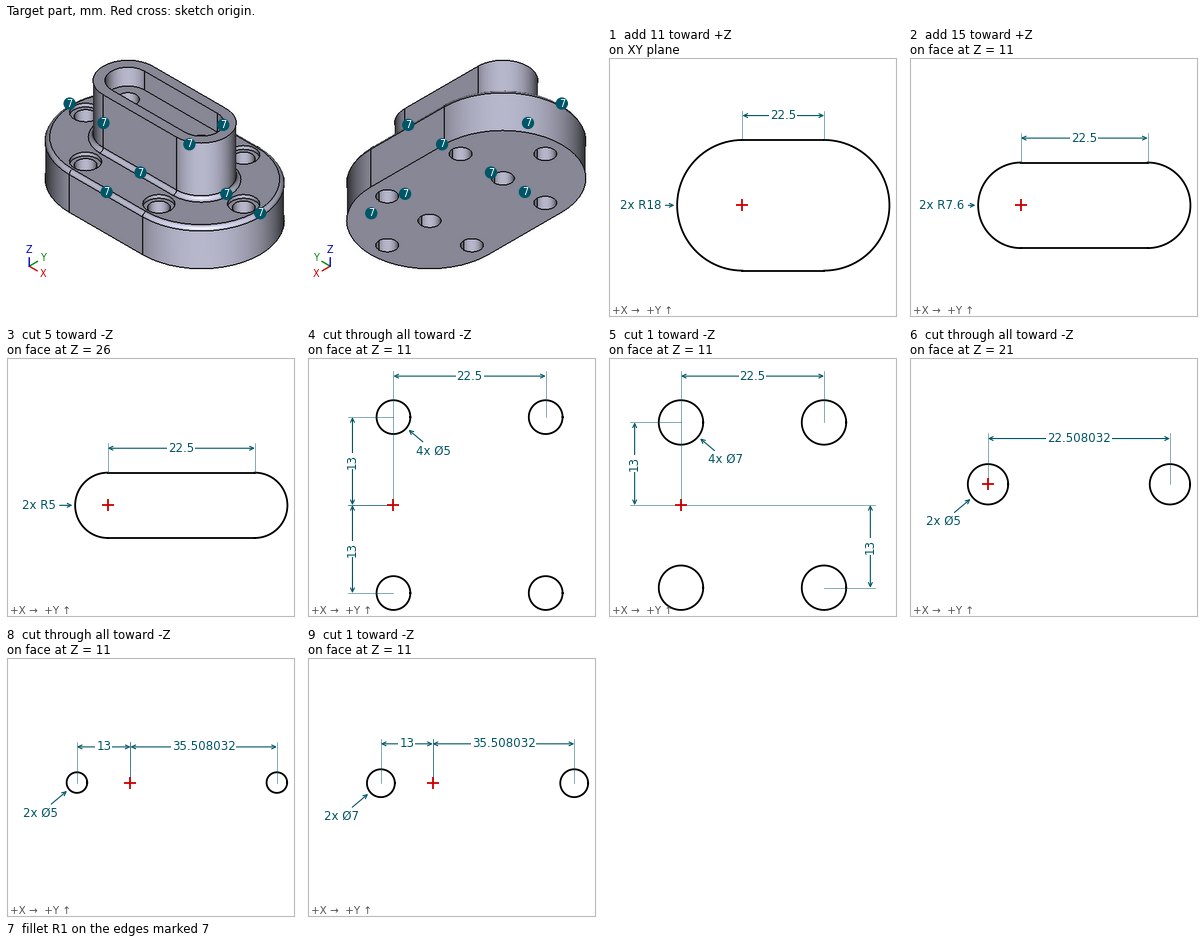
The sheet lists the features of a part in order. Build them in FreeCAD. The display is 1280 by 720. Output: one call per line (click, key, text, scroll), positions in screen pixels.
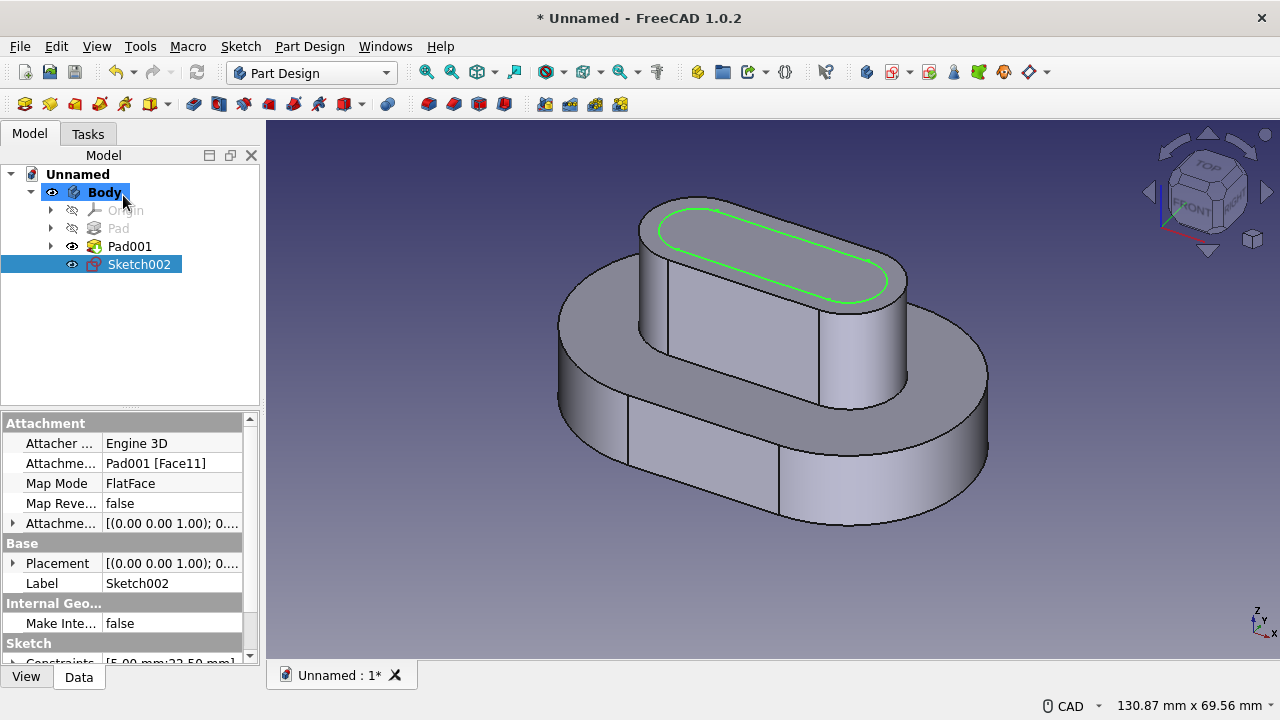
click(194, 104)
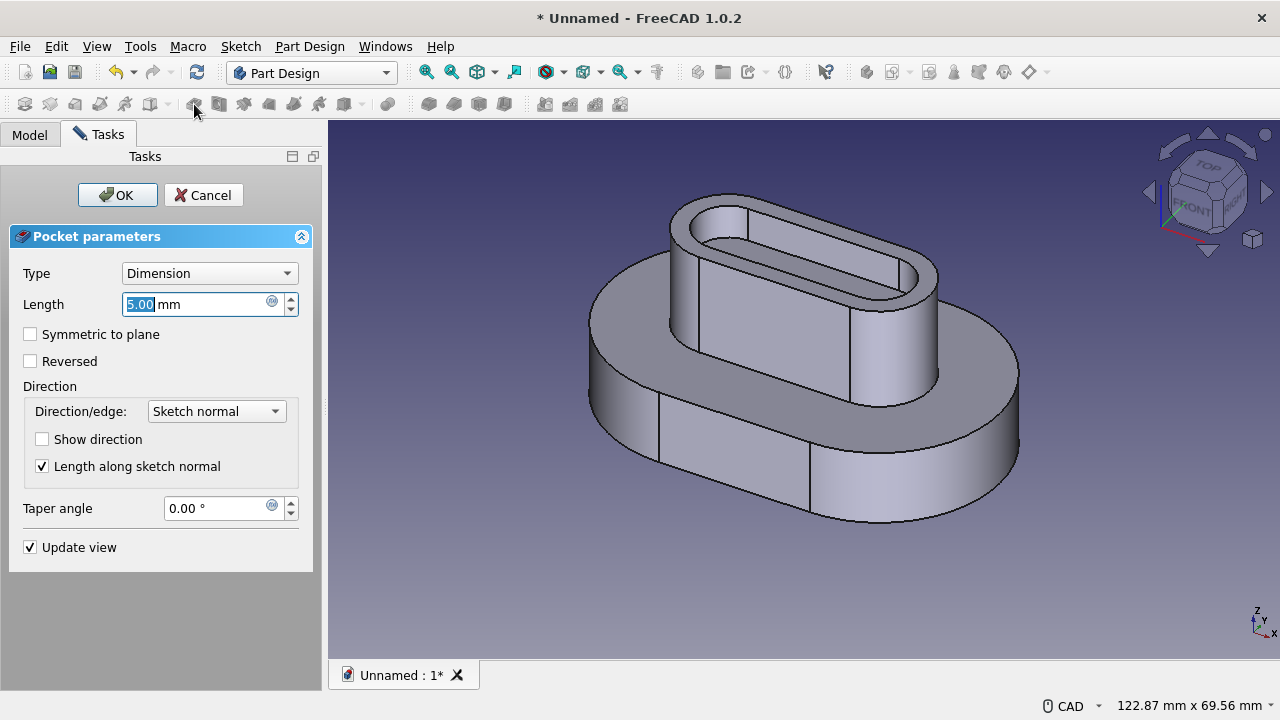
text(5)
key(Tab)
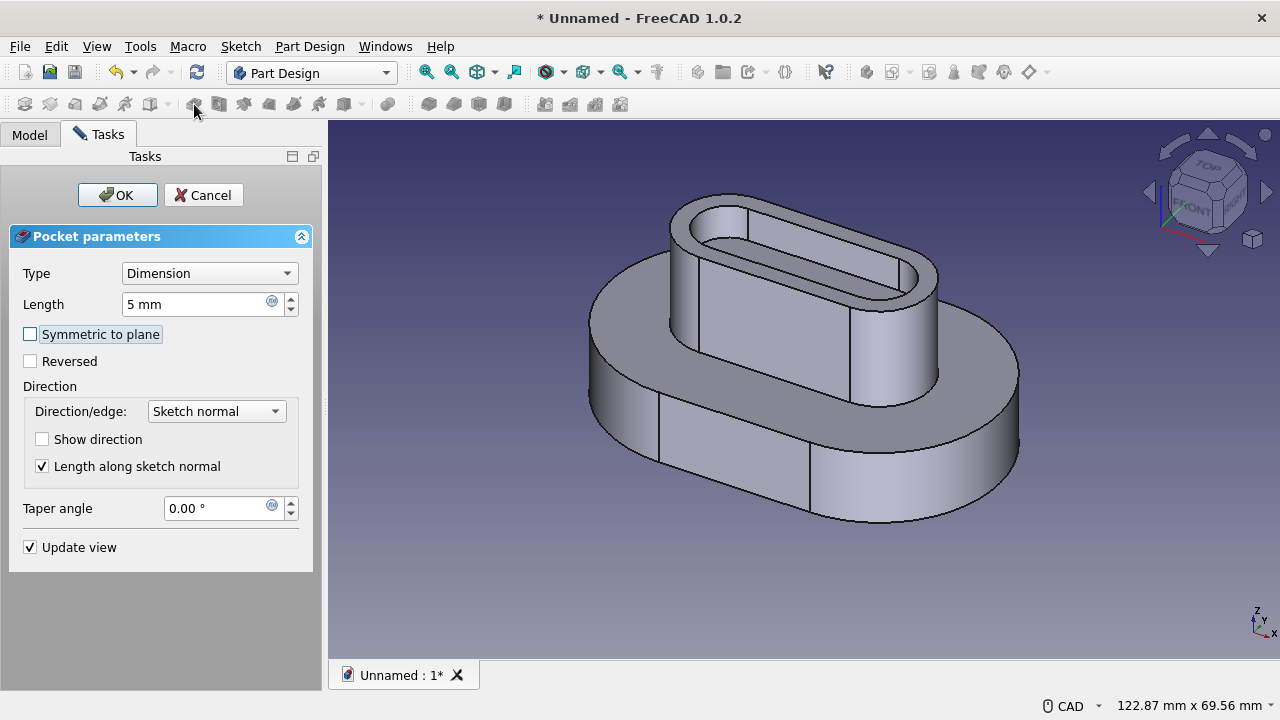
click(118, 195)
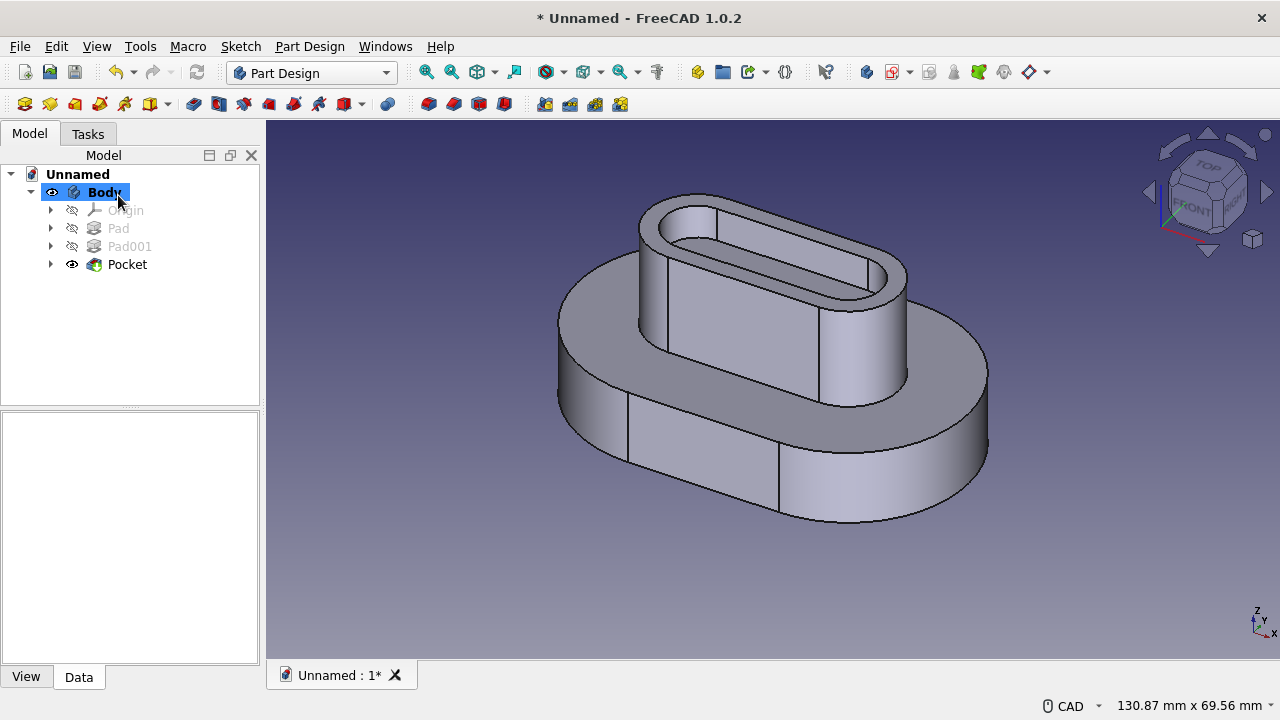
key(v)
key(f)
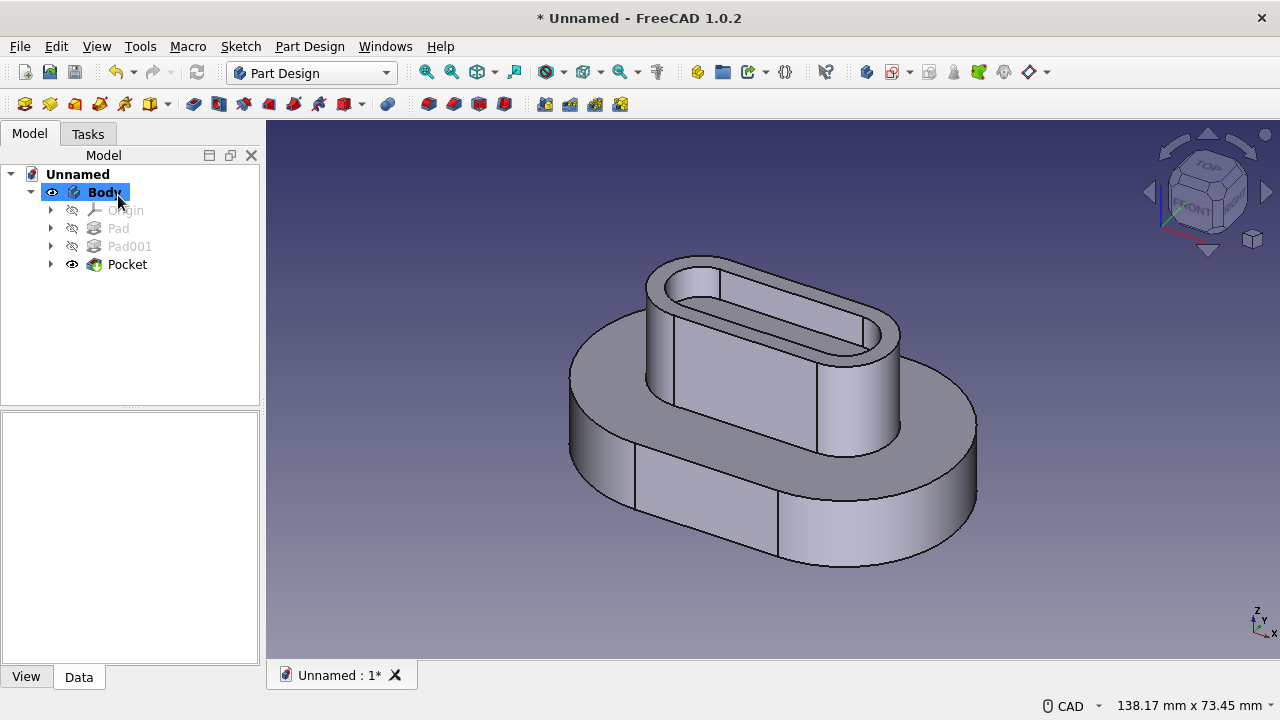
click(932, 453)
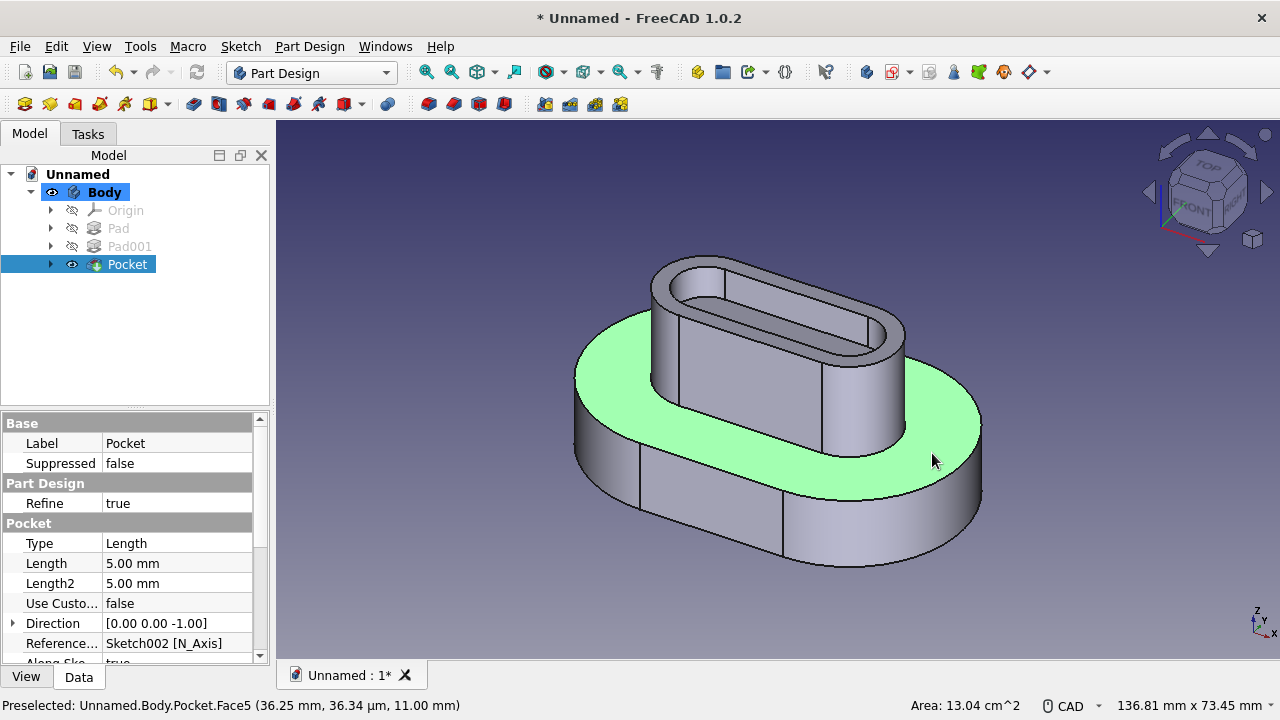
click(892, 72)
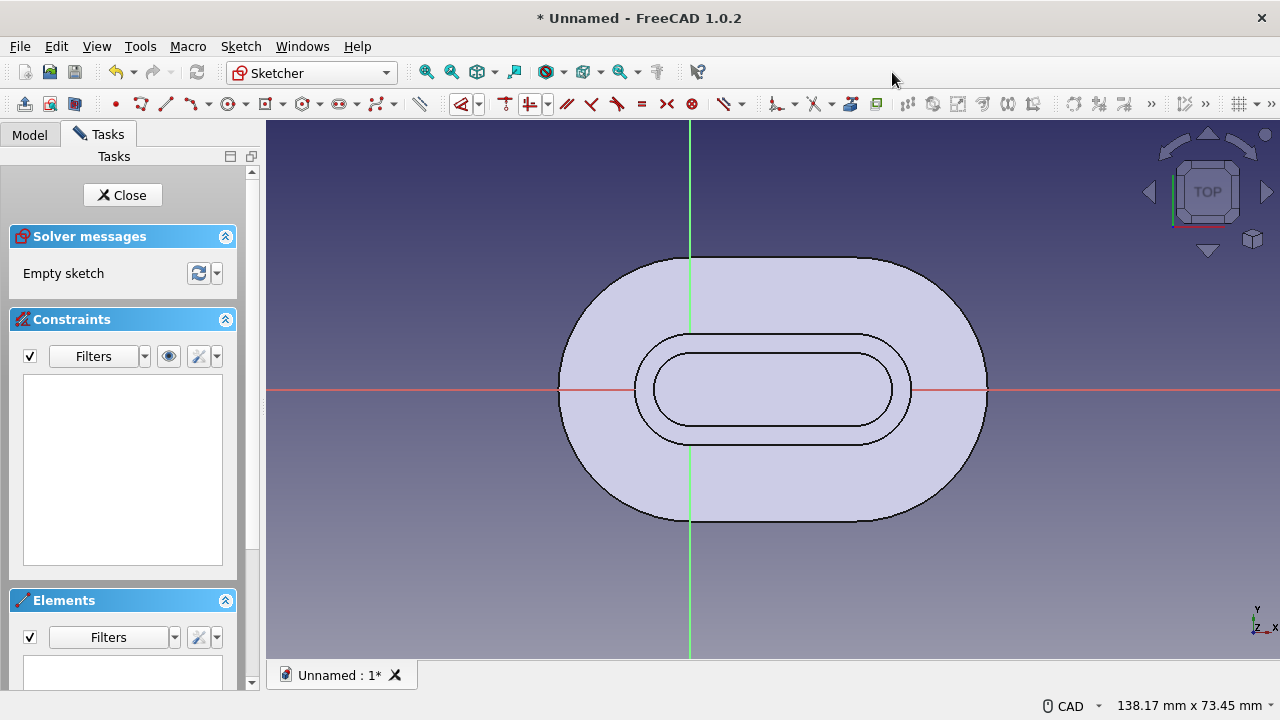
scroll(912, 390, up, 2)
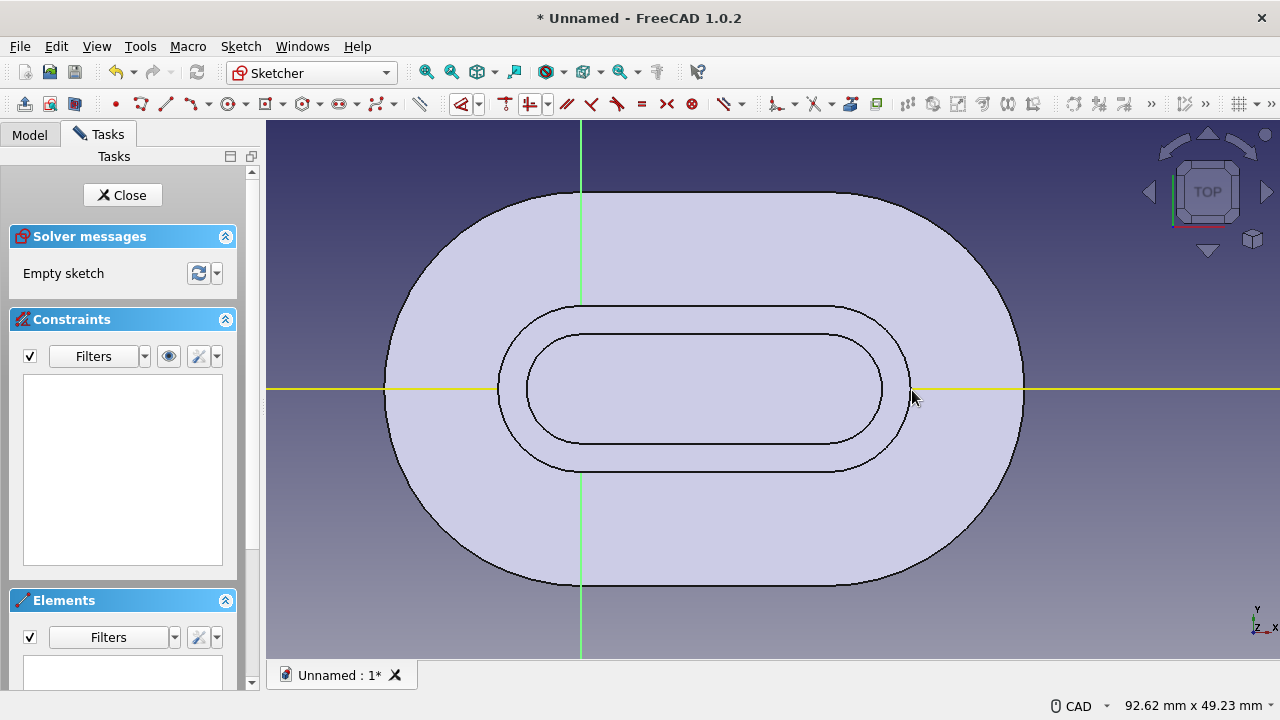
key(g)
key(c)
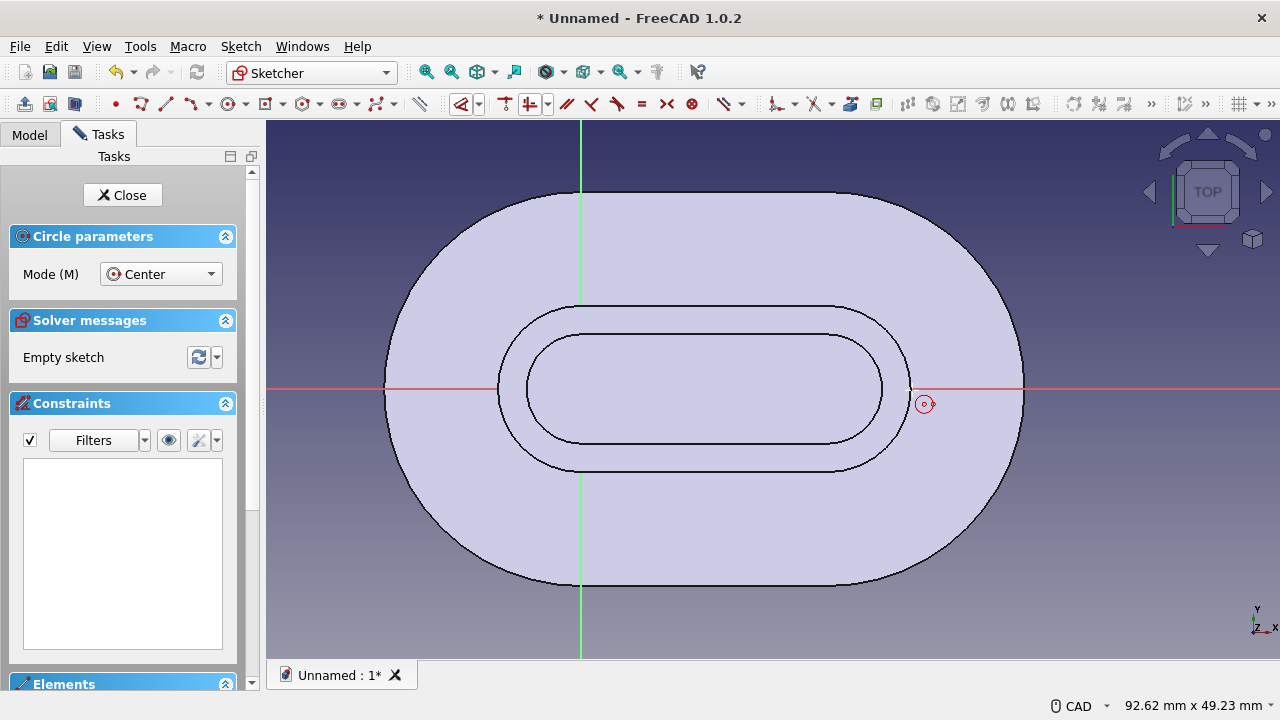
click(581, 247)
move(601, 227)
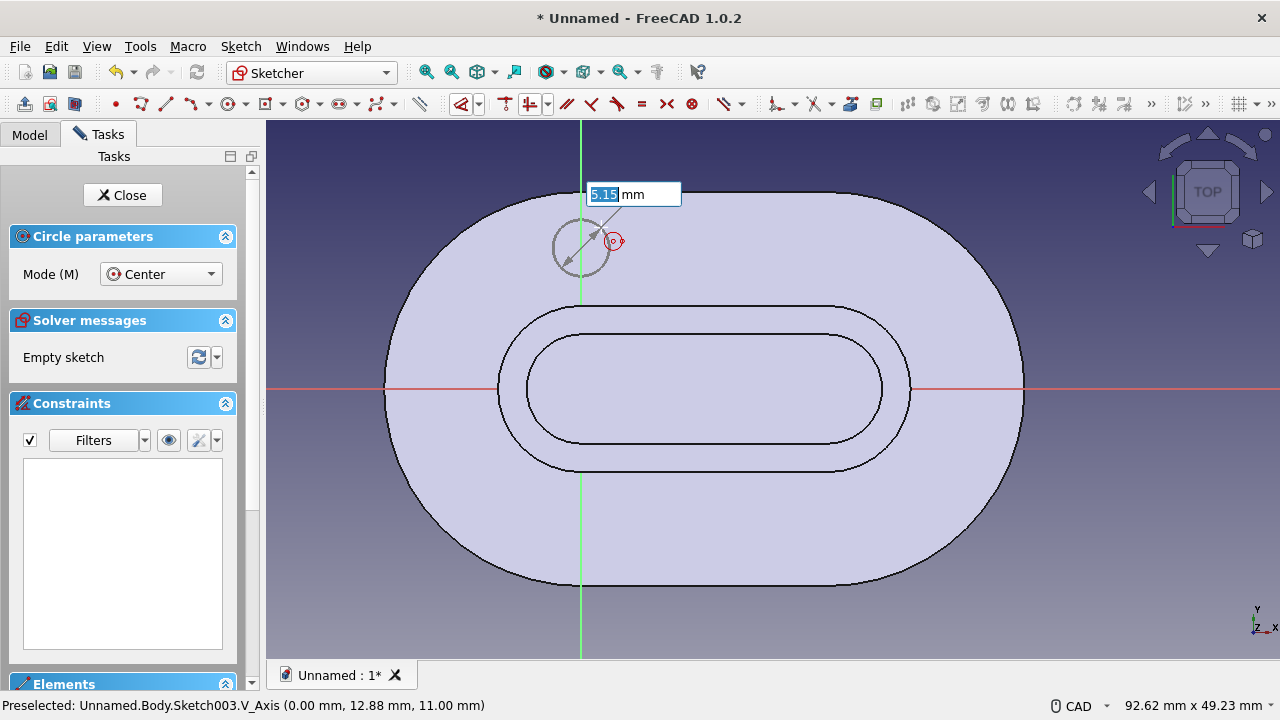
text(5)
key(Return)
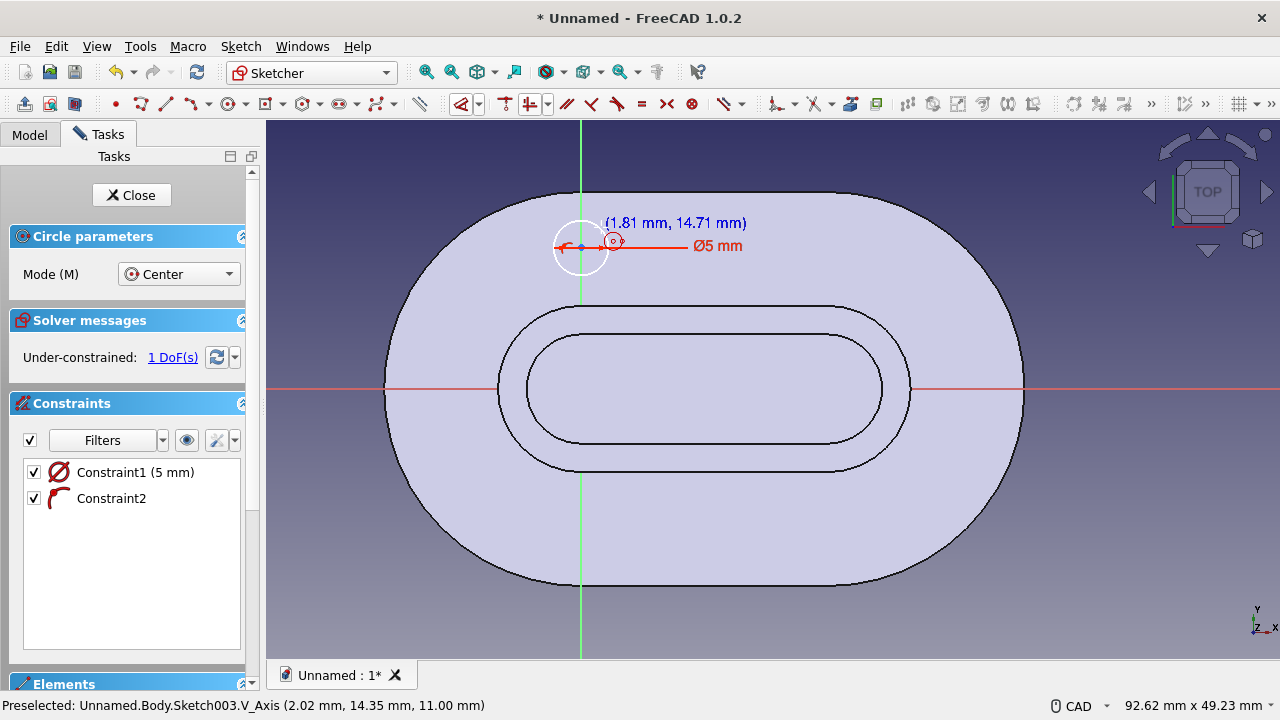
click(827, 247)
move(847, 227)